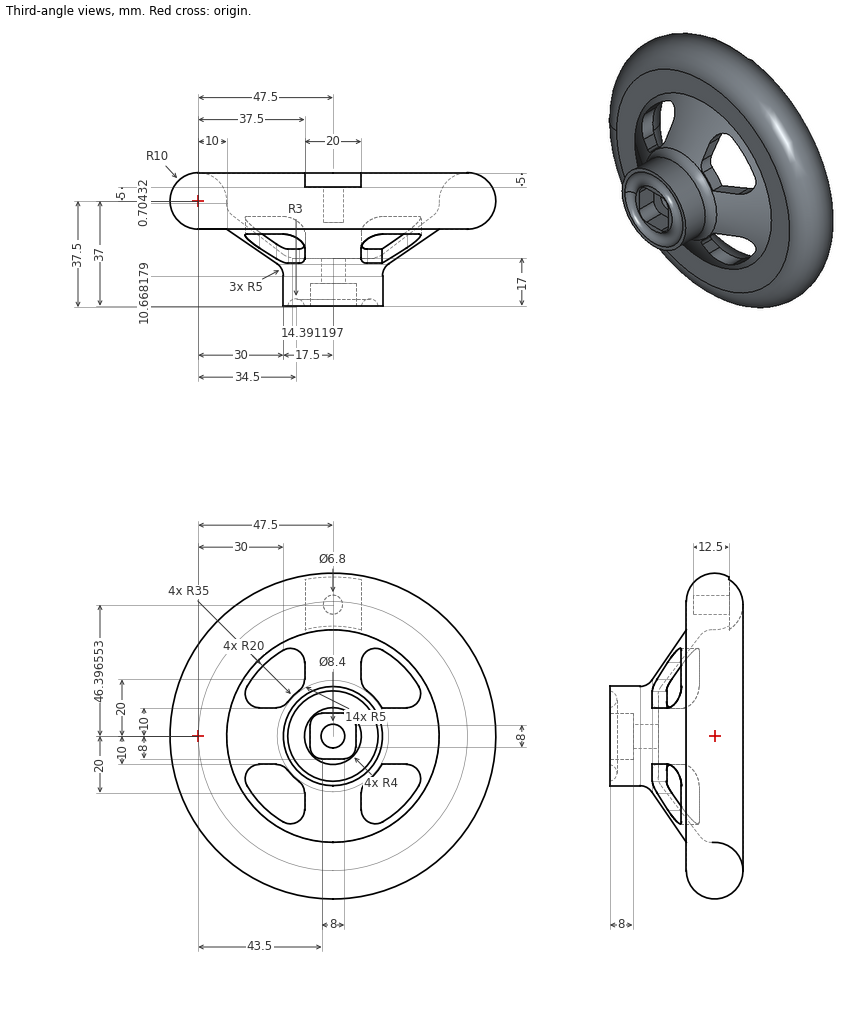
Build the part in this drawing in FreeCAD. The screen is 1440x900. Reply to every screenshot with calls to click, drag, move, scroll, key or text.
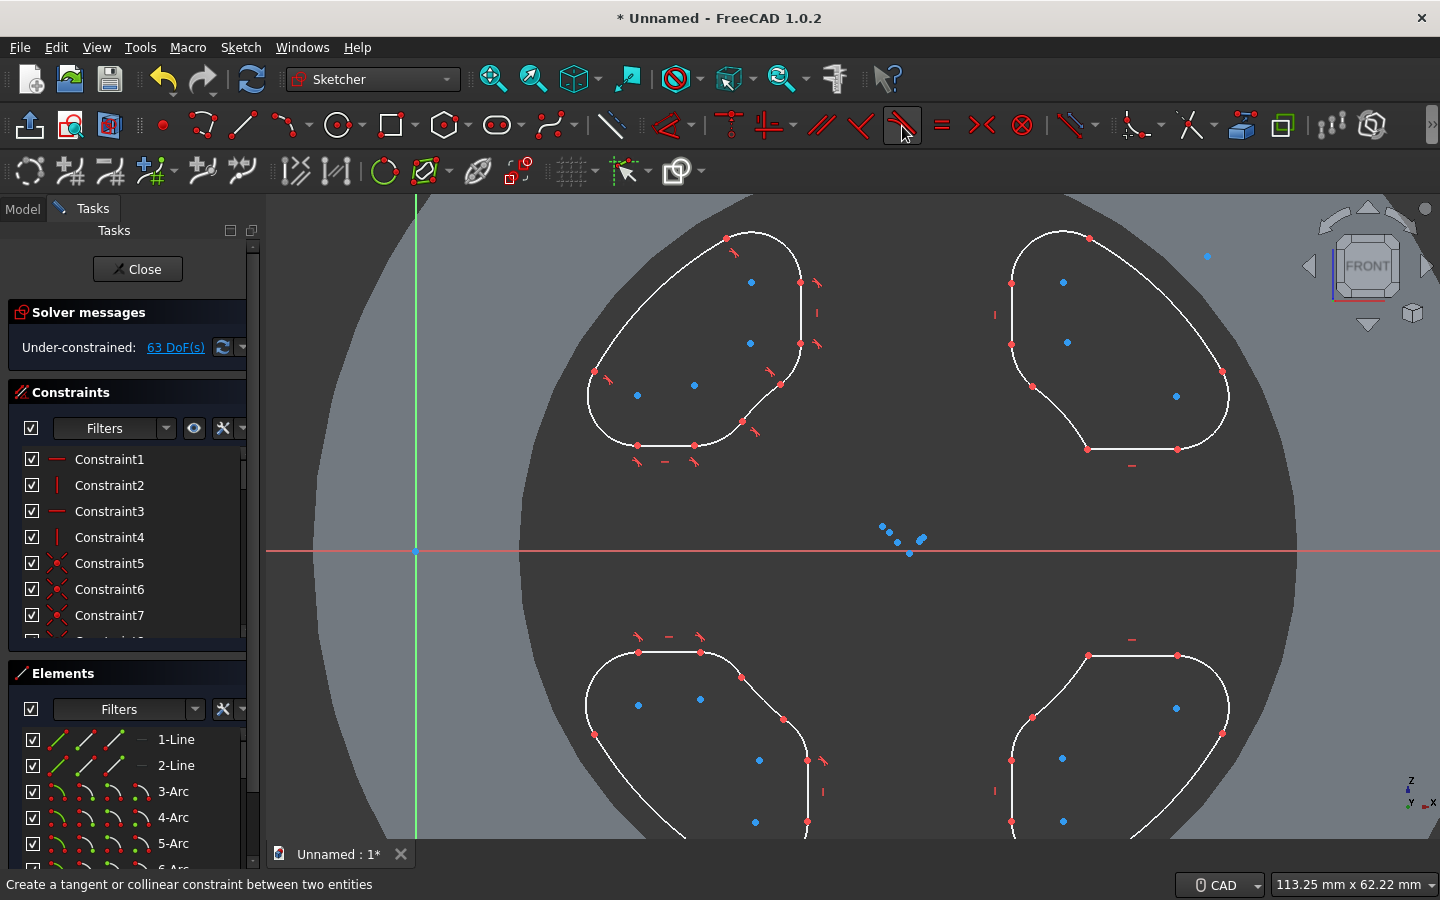
click(808, 779)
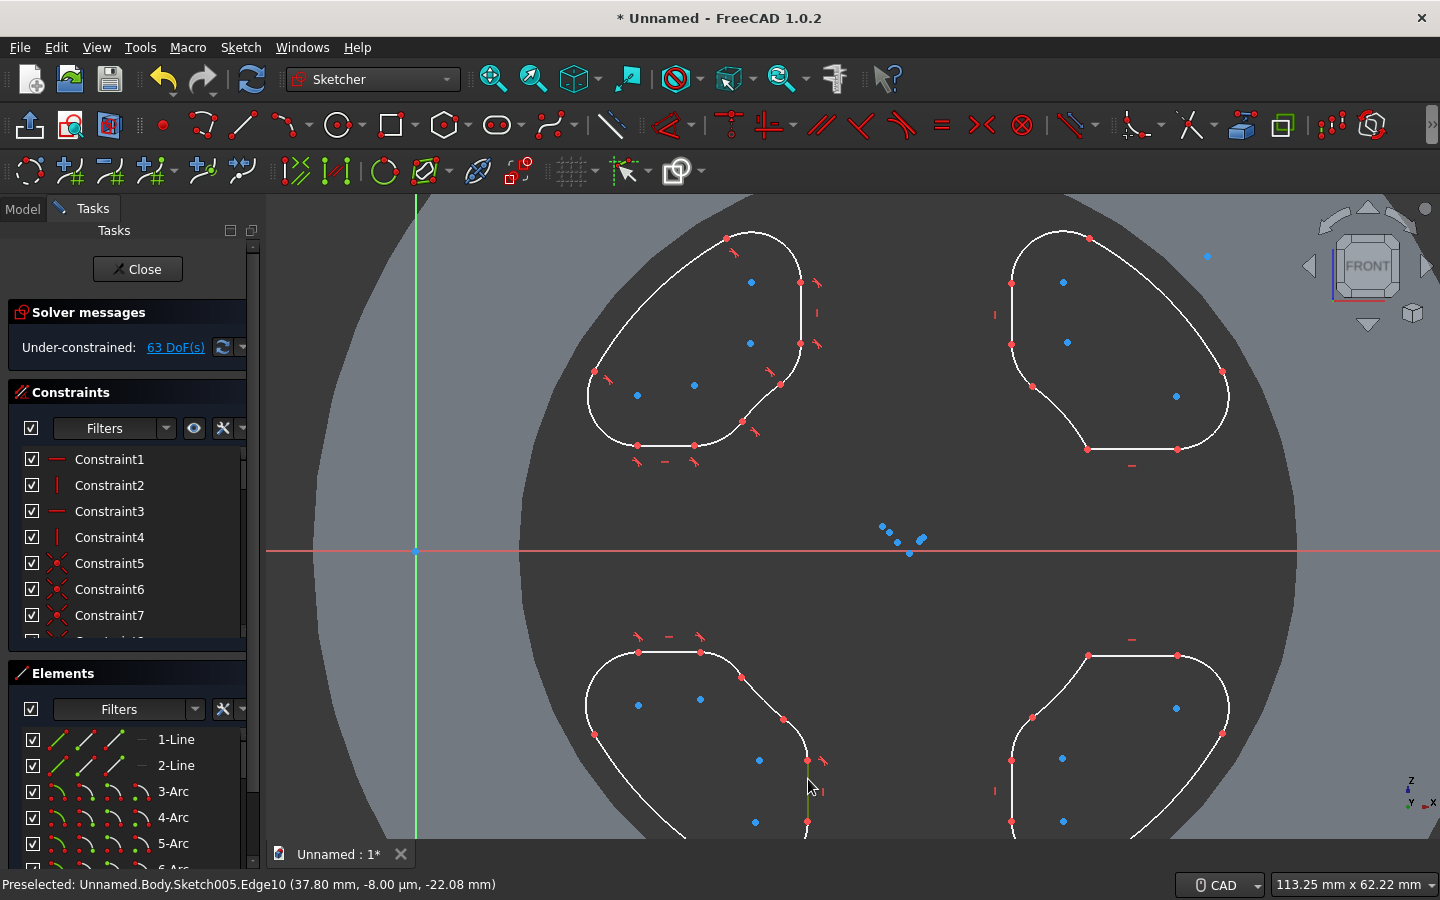
scroll(714, 446, down, 2)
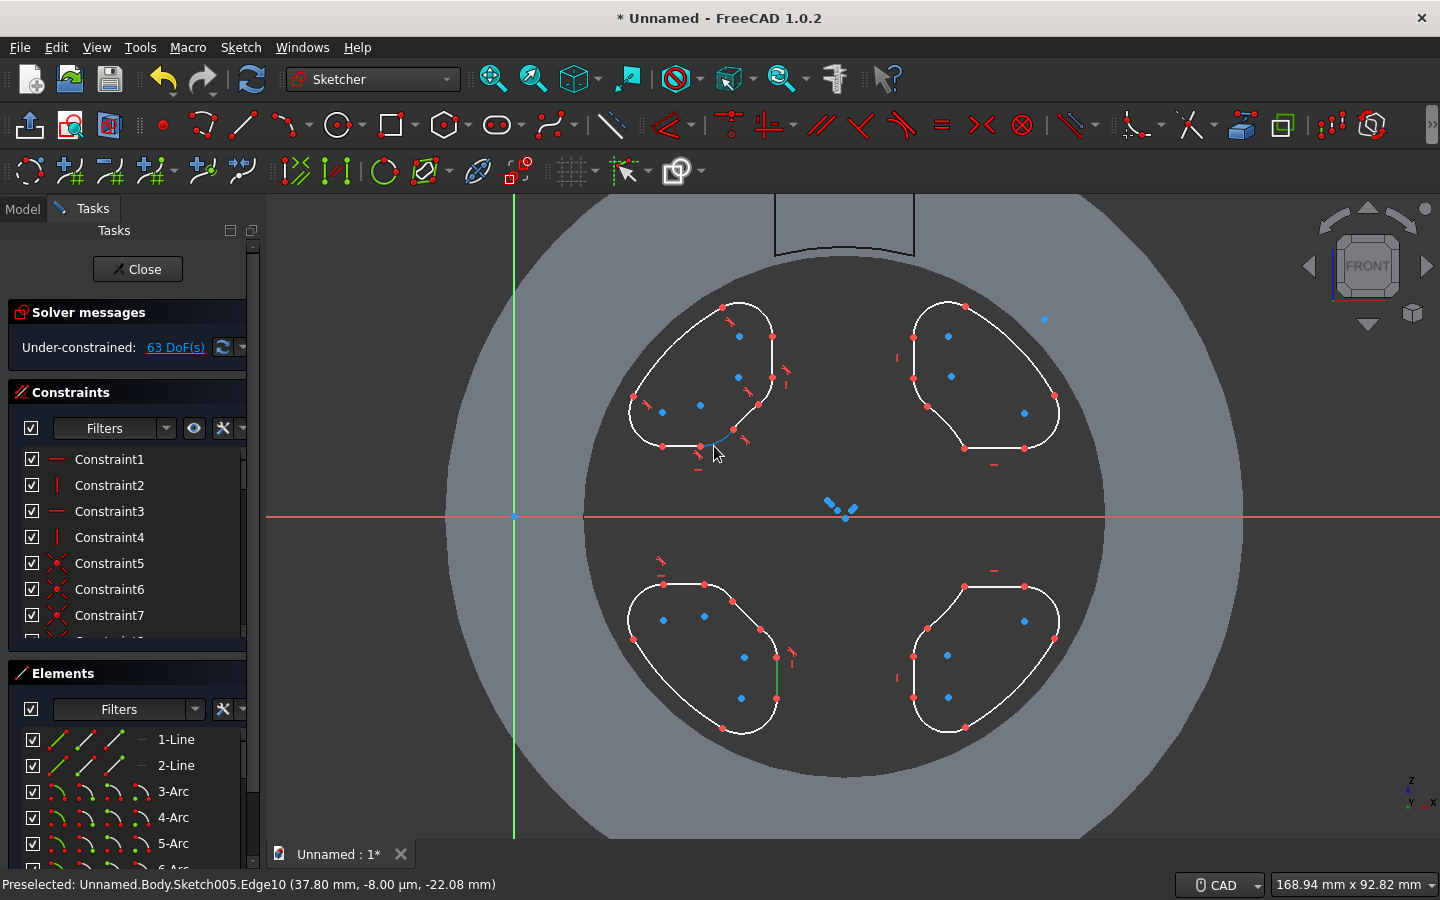
click(744, 734)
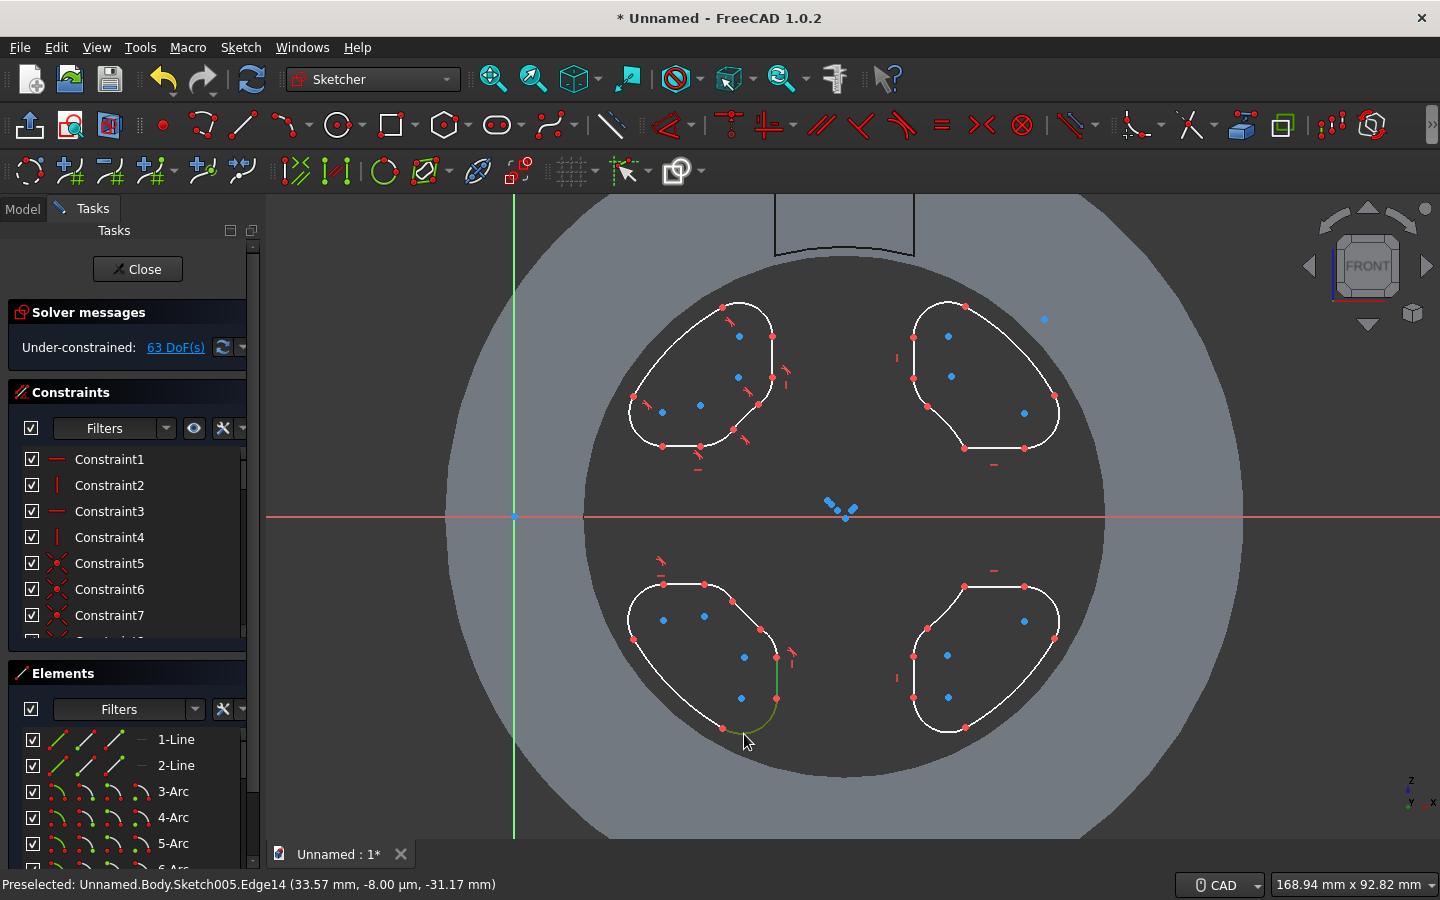
click(902, 126)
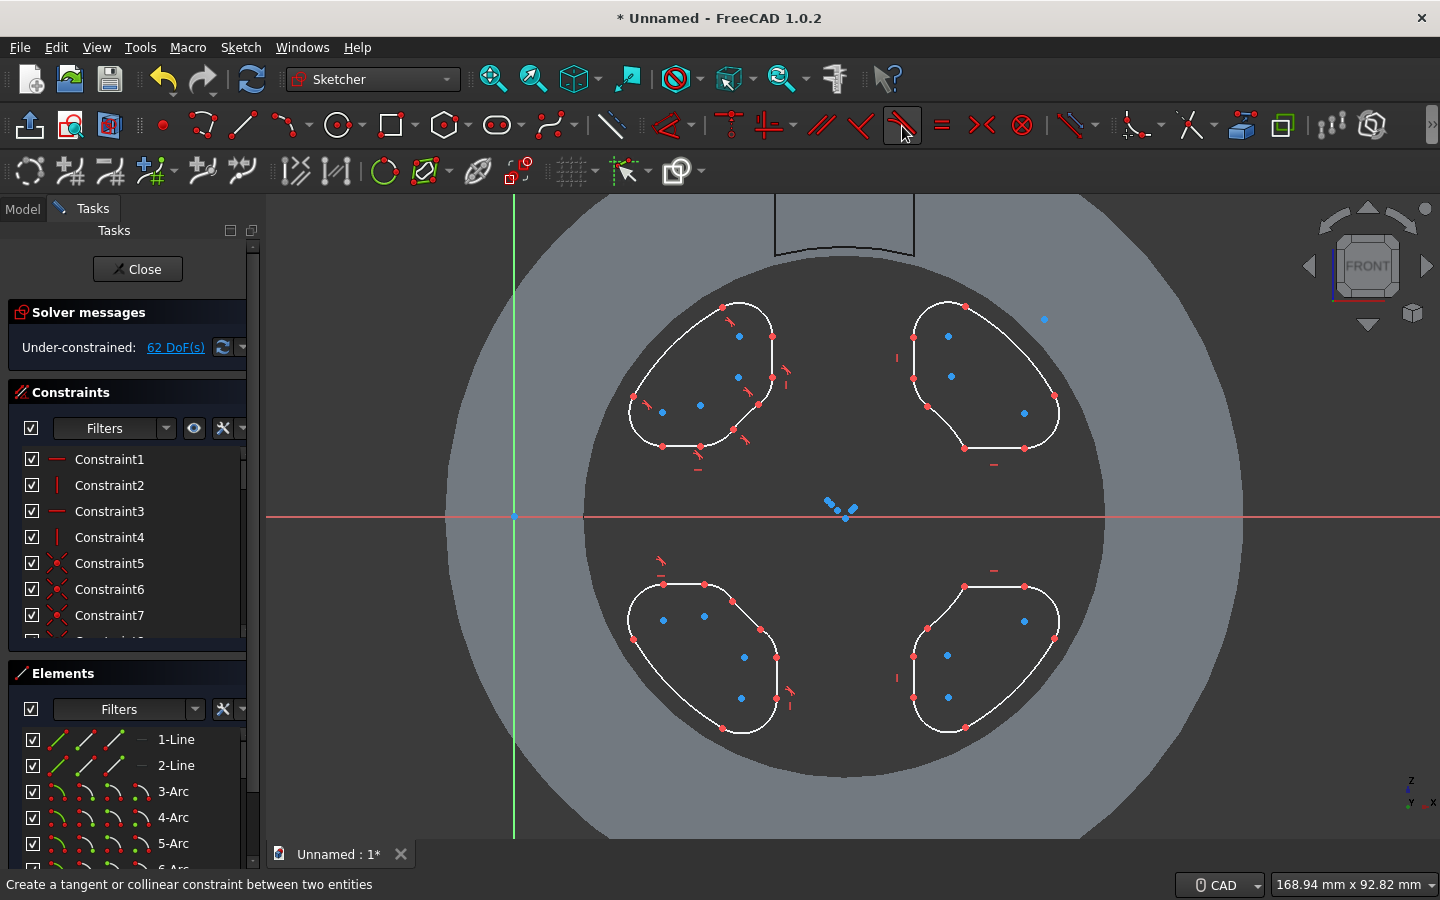
scroll(727, 593, up, 2)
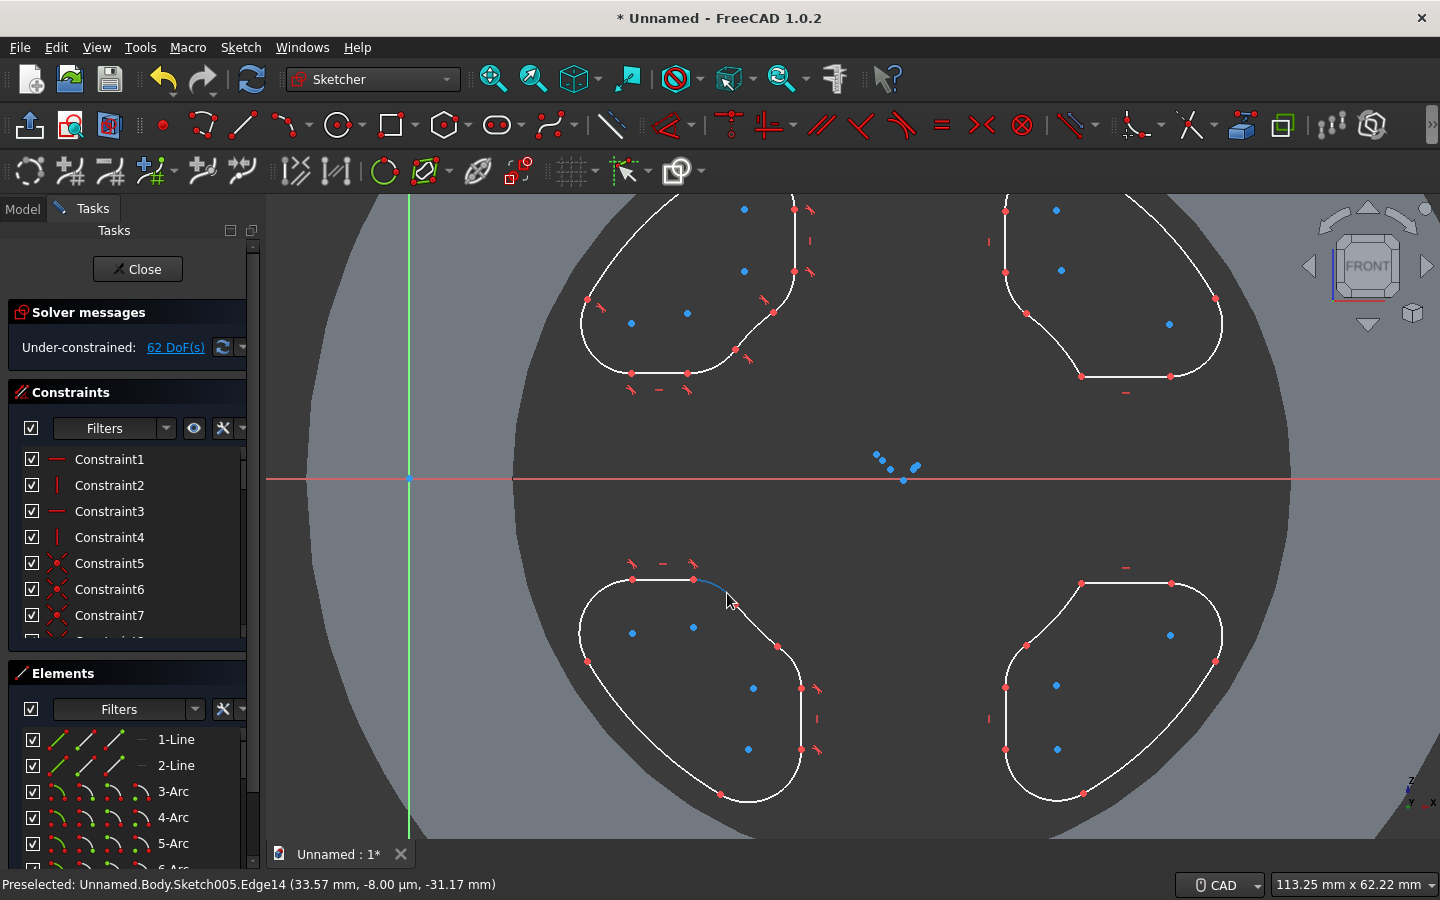
click(726, 593)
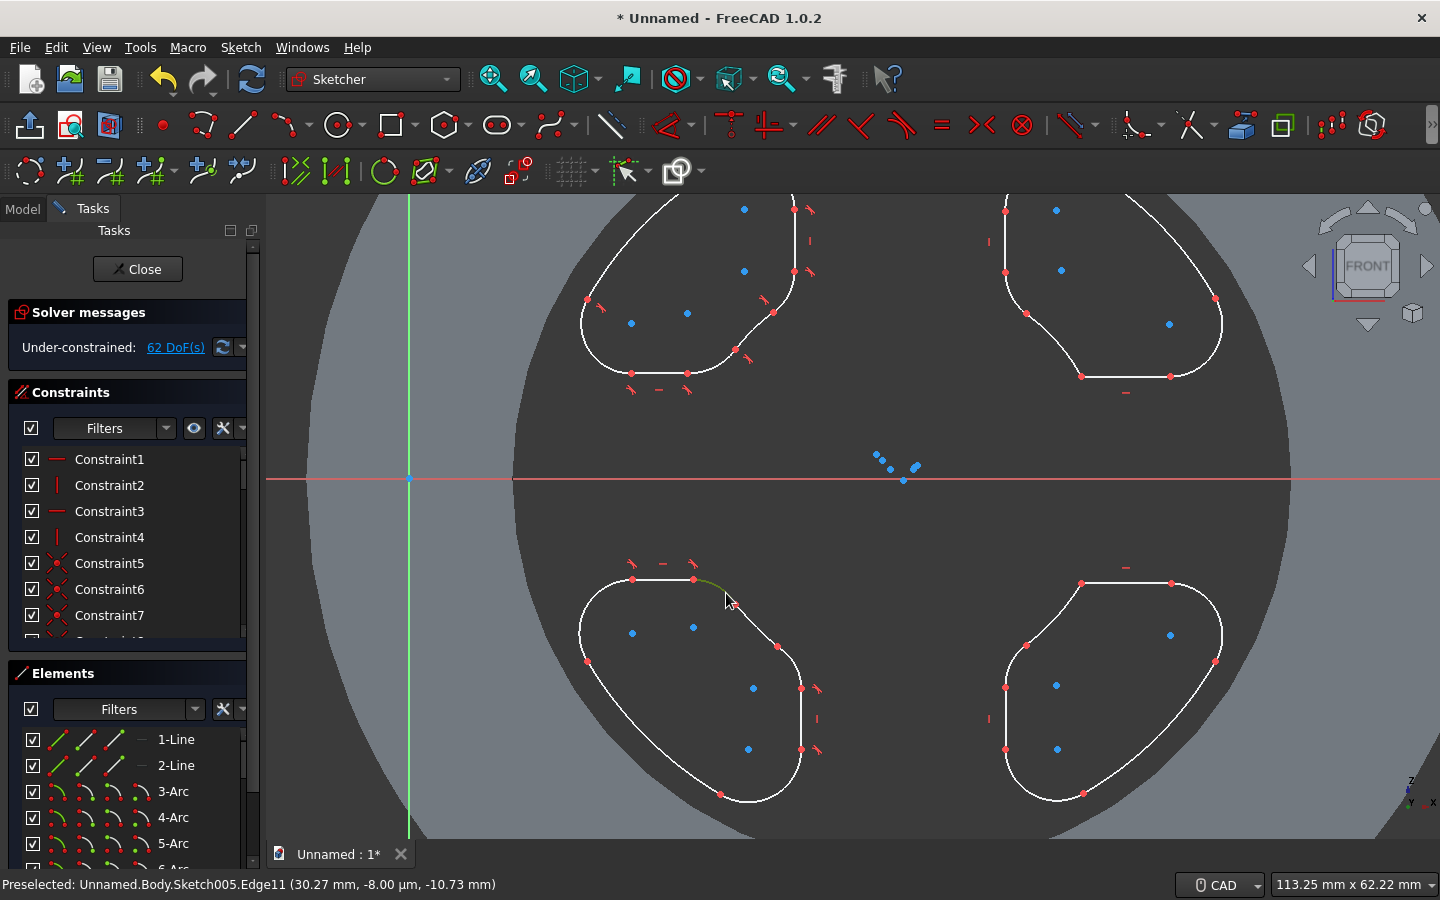
click(748, 618)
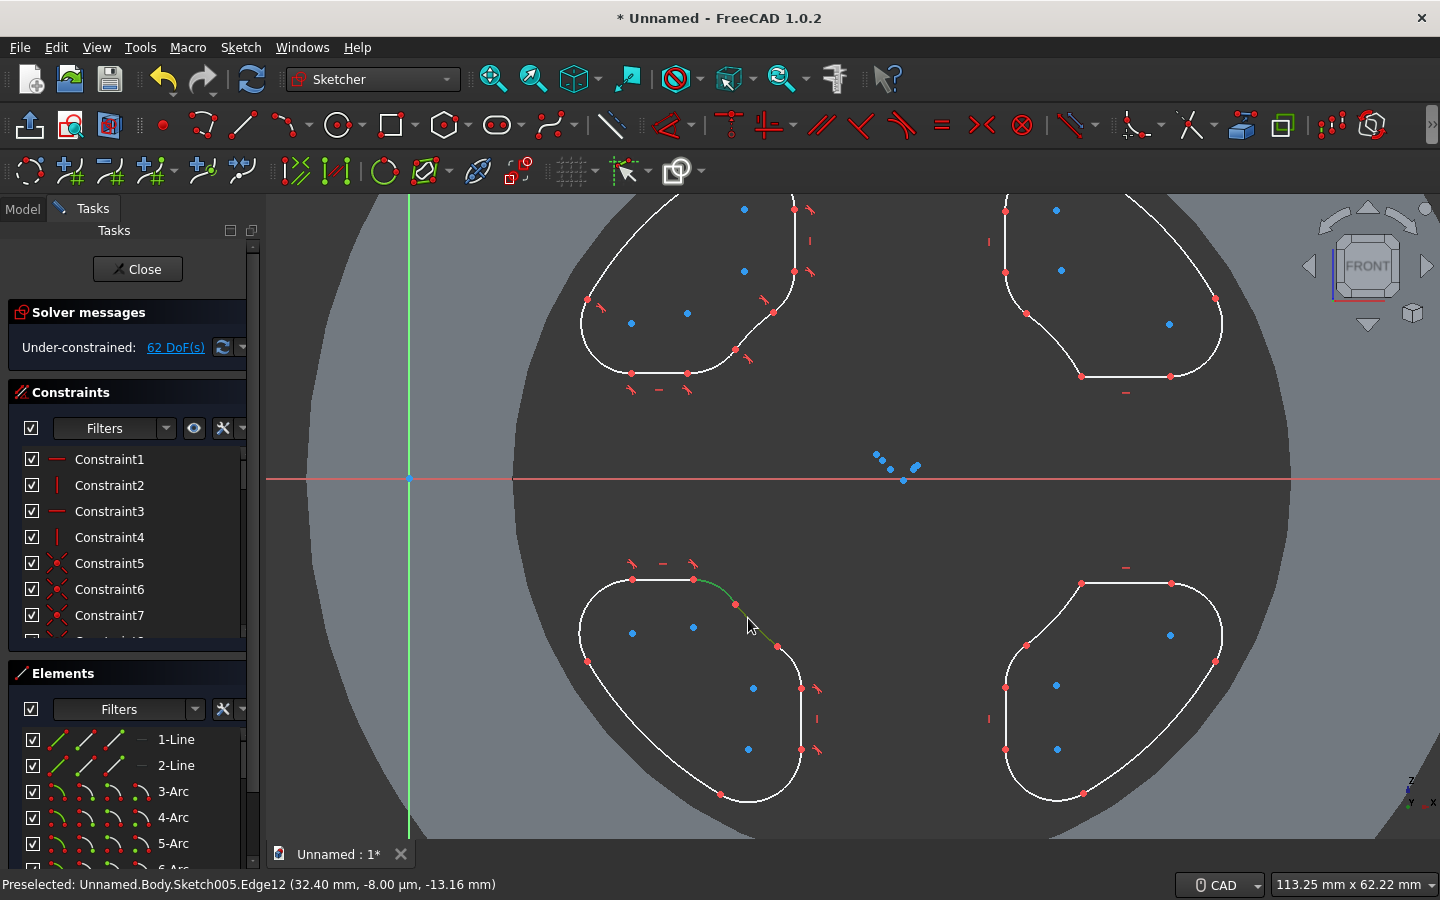
click(902, 126)